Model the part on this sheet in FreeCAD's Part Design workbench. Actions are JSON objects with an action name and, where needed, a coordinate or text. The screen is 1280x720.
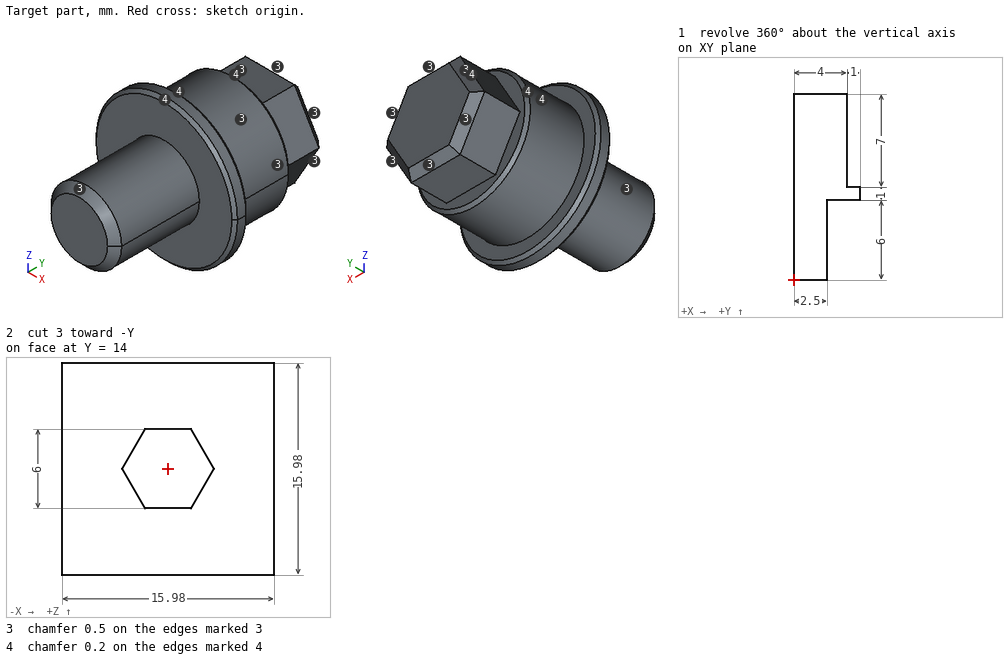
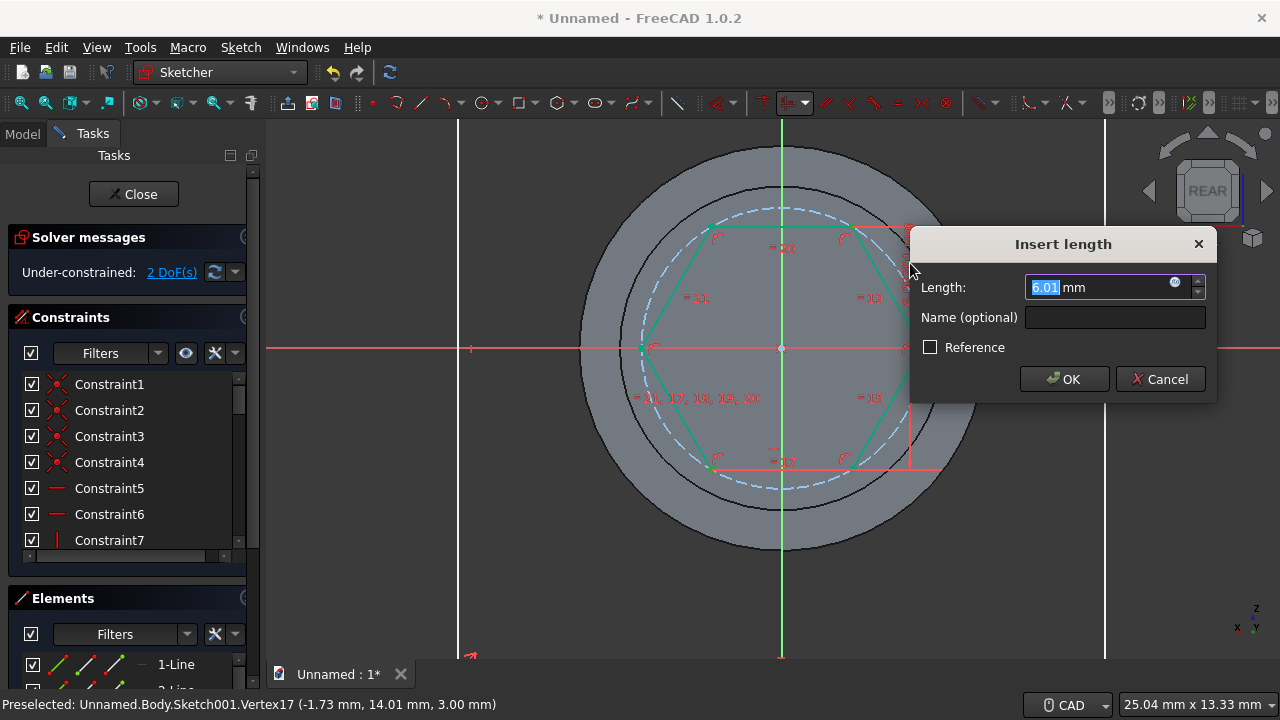
{"action": "type", "text": "6"}
{"action": "key", "text": "Return"}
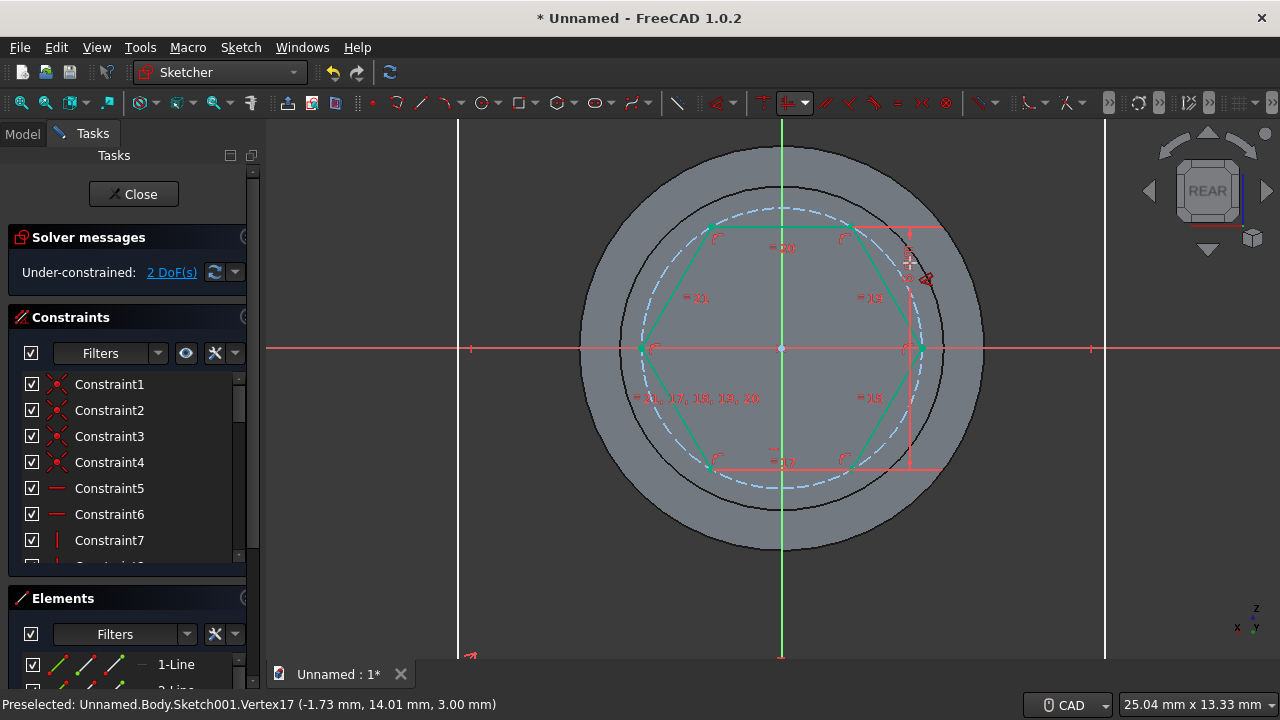
{"action": "scroll", "coordinate": [610, 438], "scroll_direction": "down", "scroll_amount": 3}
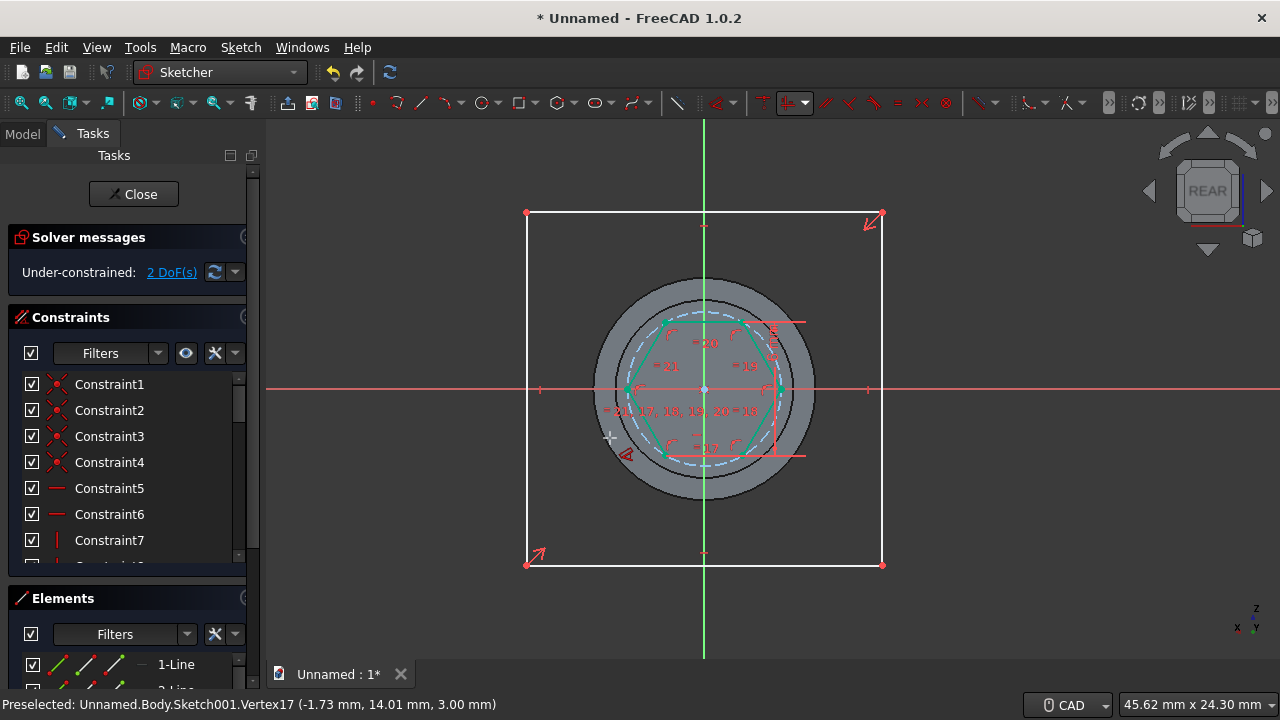
{"action": "left_click", "coordinate": [633, 566]}
{"action": "left_click", "coordinate": [623, 600]}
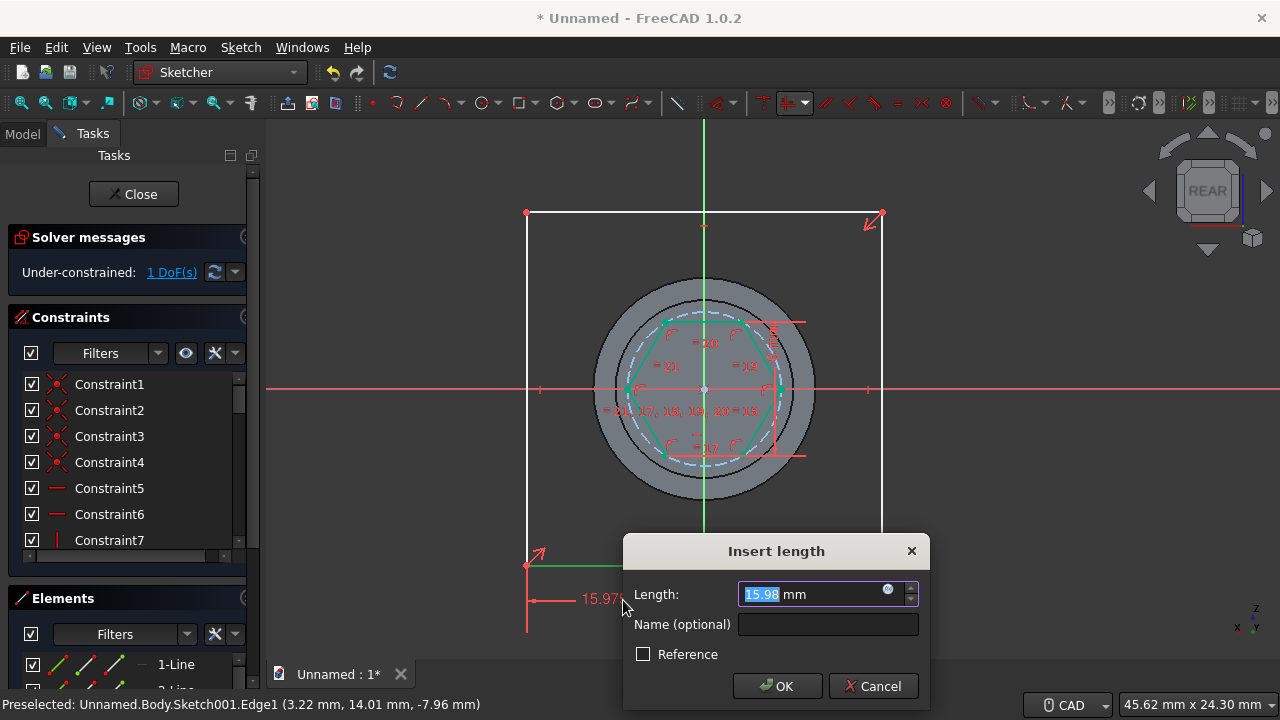
{"action": "type", "text": "15.98"}
{"action": "key", "text": "Return"}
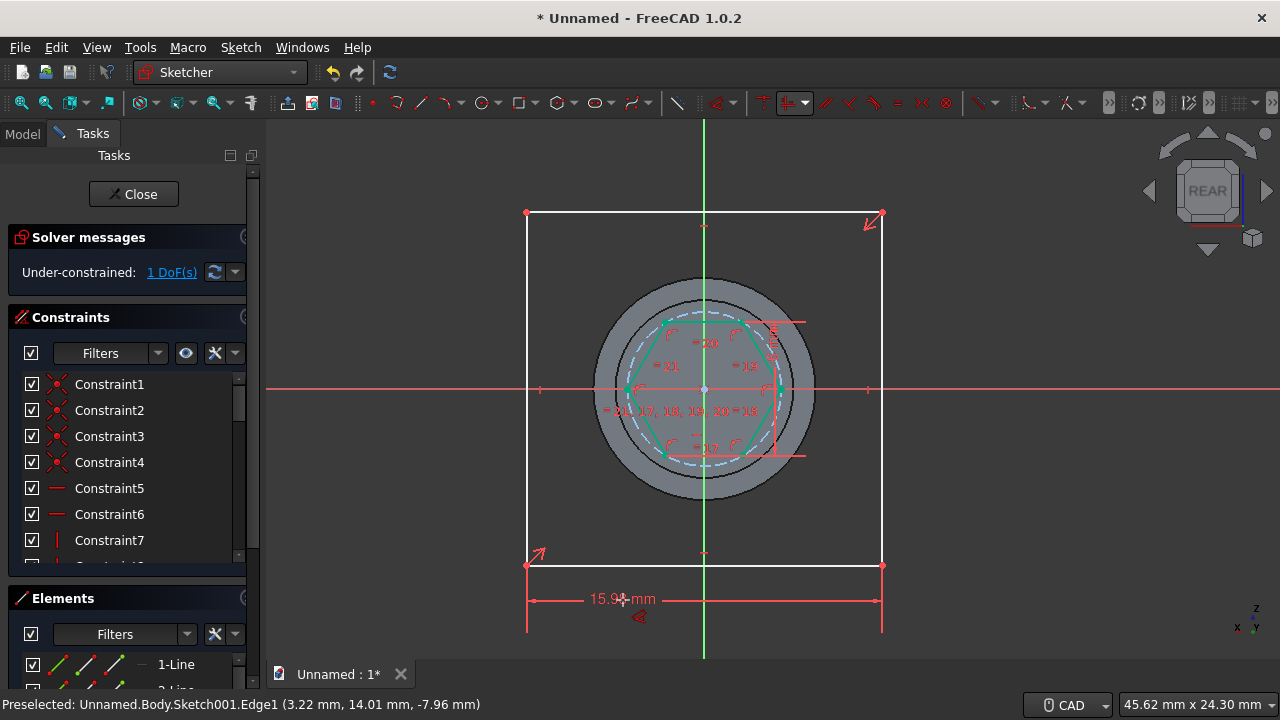
{"action": "left_click", "coordinate": [882, 460]}
{"action": "left_click", "coordinate": [916, 308]}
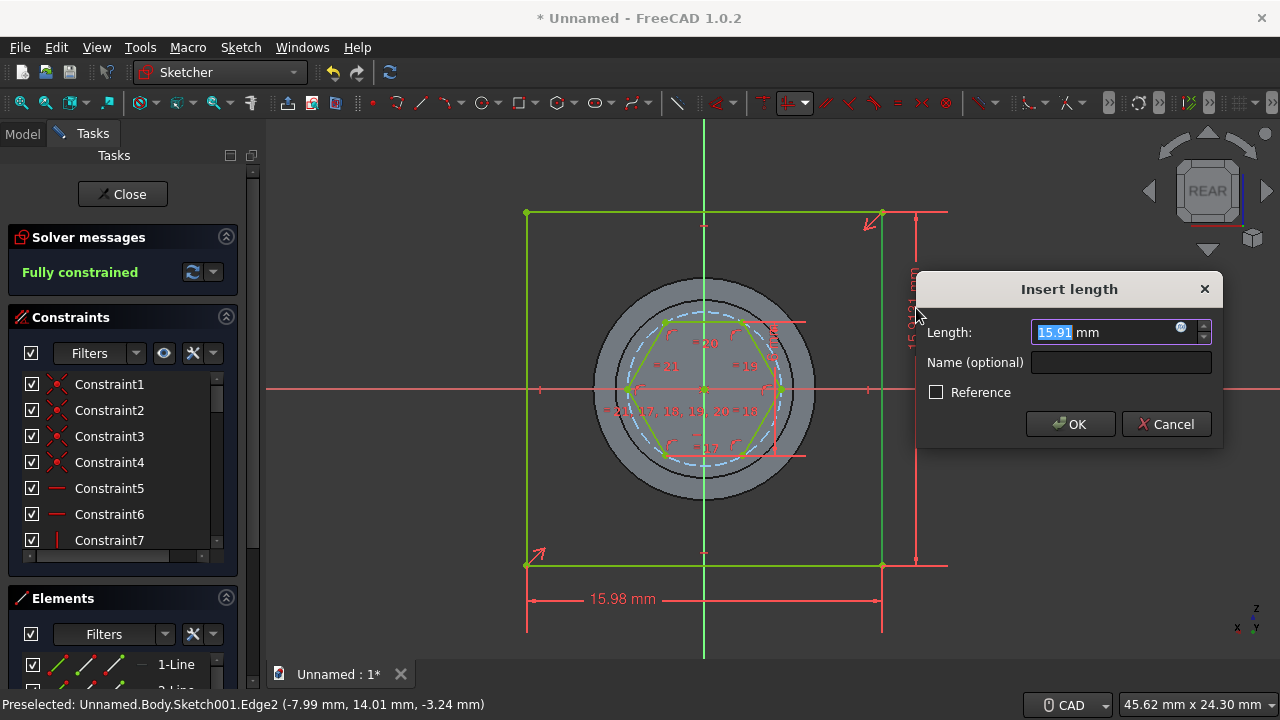
{"action": "type", "text": "15.98"}
{"action": "key", "text": "Return"}
{"action": "key", "text": "Escape"}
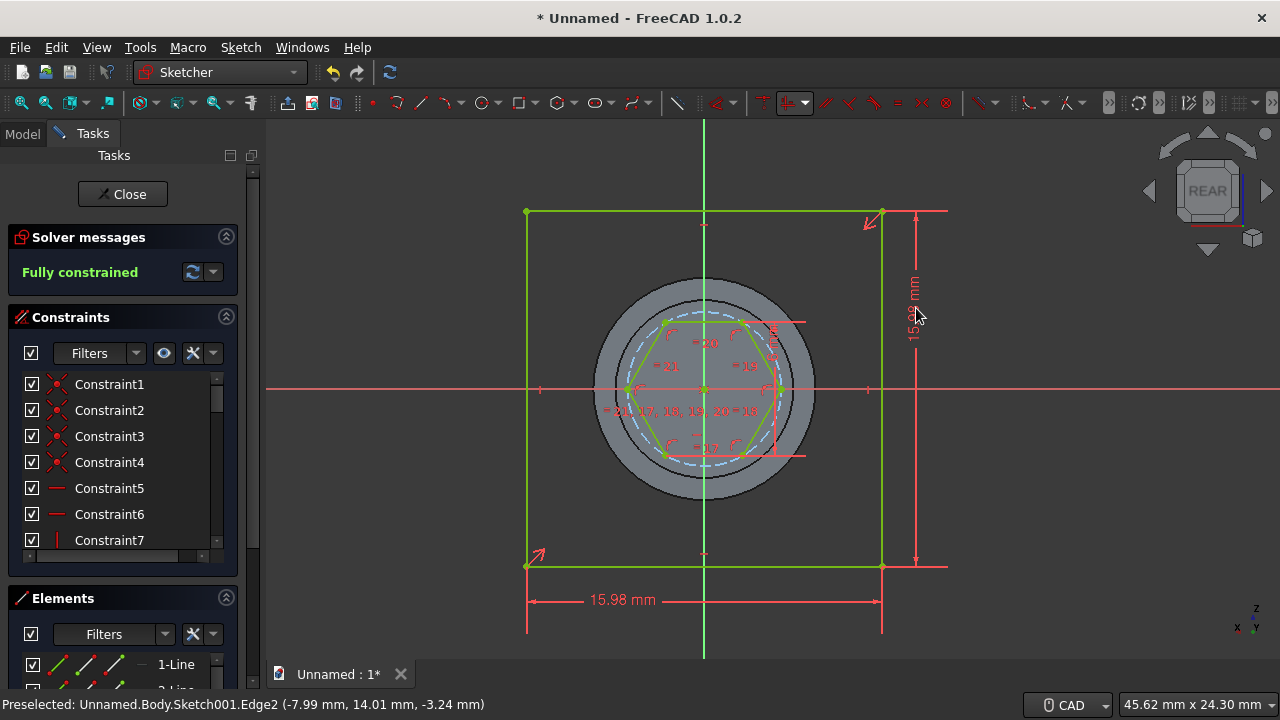
{"action": "left_click", "coordinate": [123, 194]}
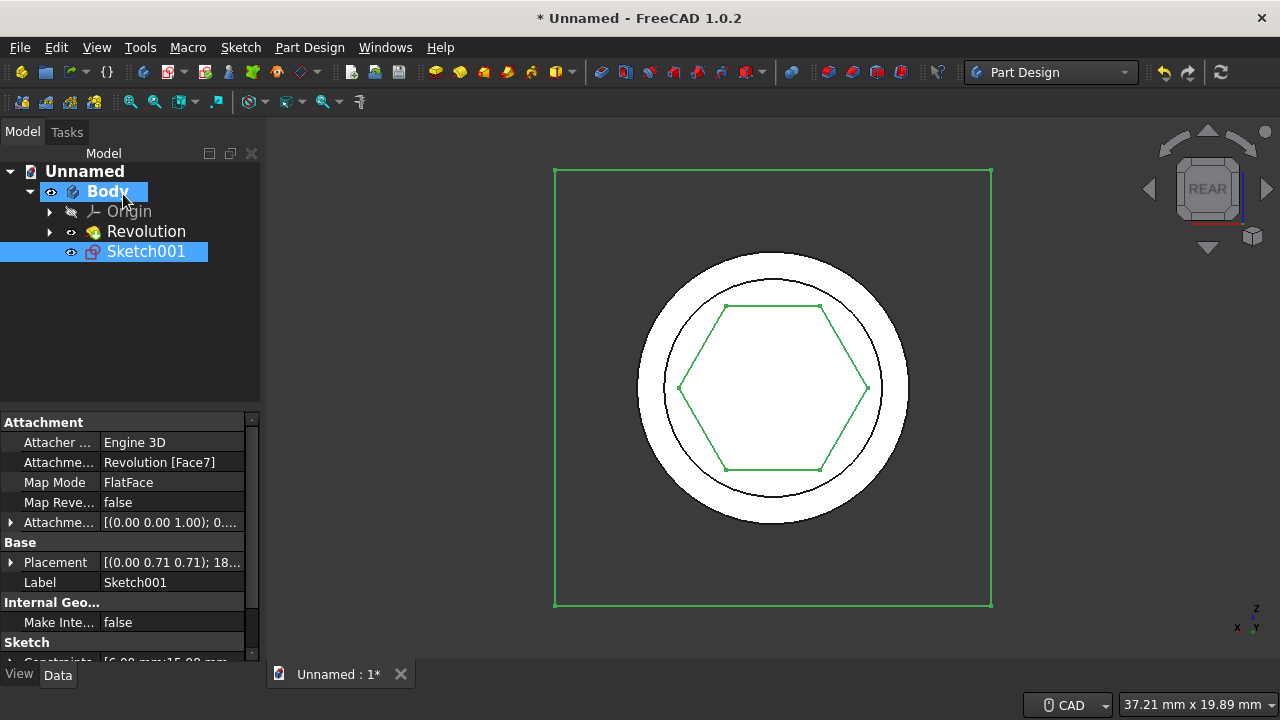
{"action": "left_click", "coordinate": [602, 72]}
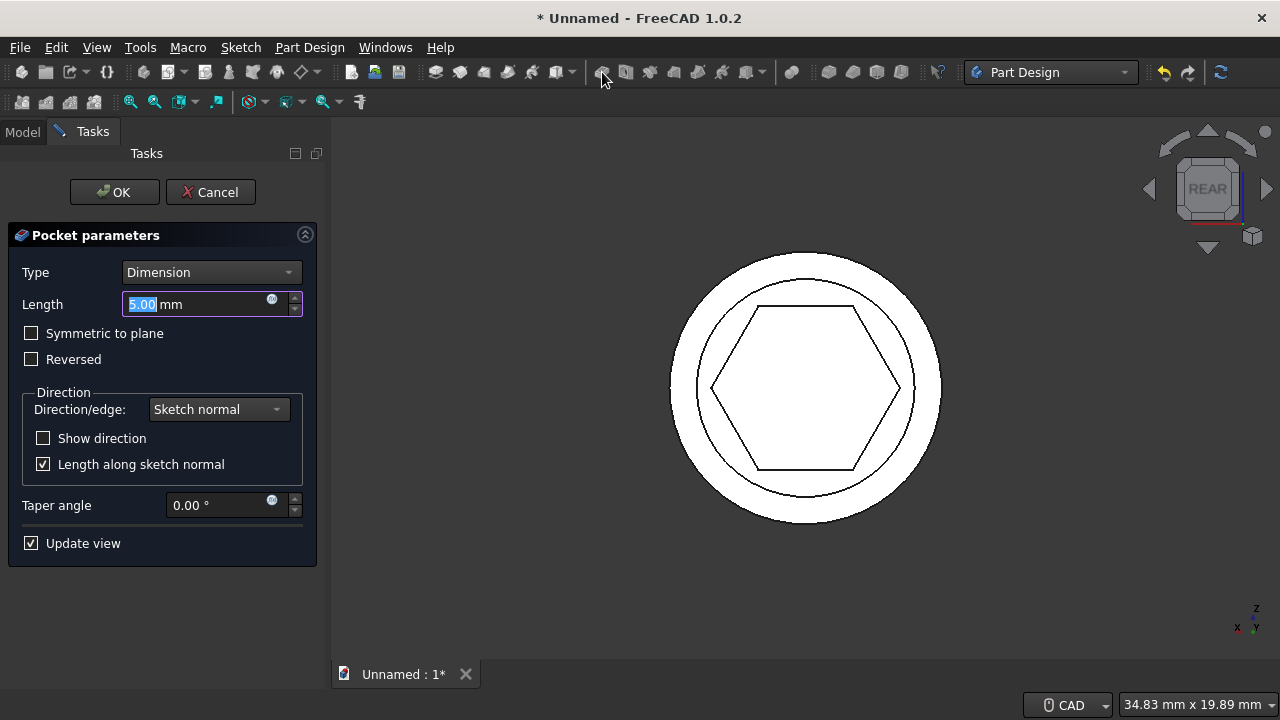
{"action": "type", "text": "3"}
{"action": "key", "text": "Tab"}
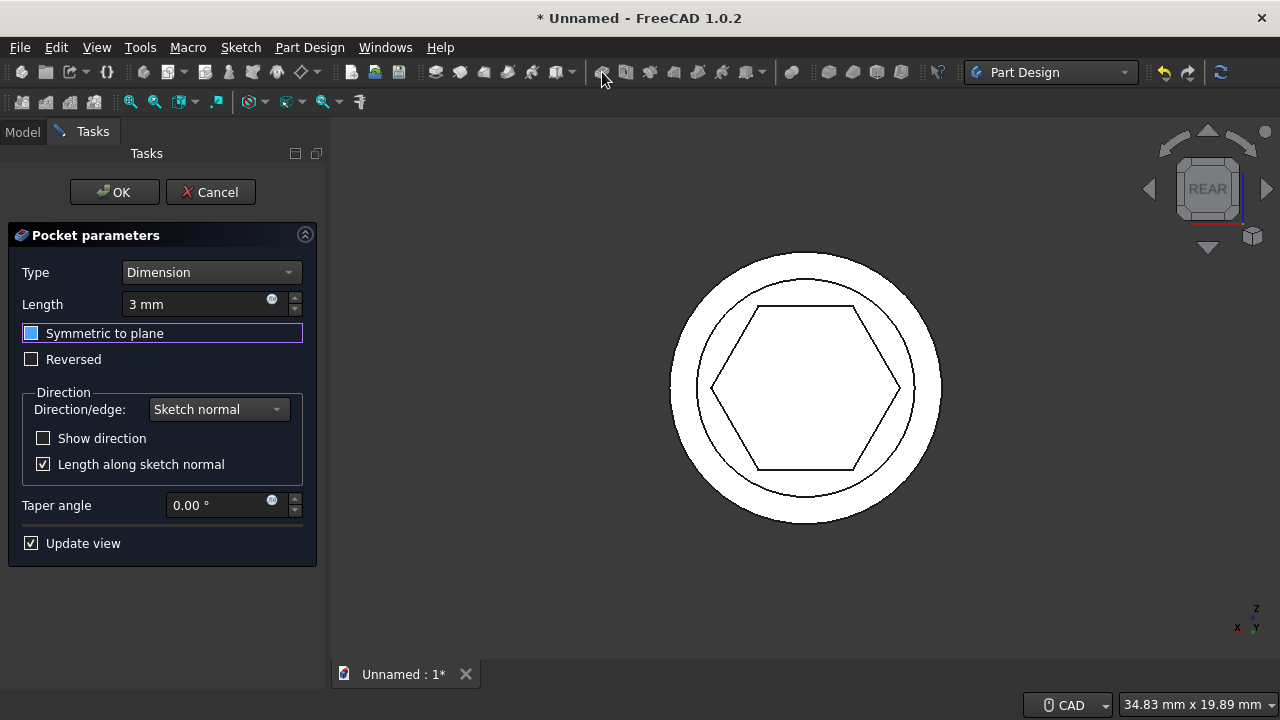
{"action": "left_click", "coordinate": [115, 192]}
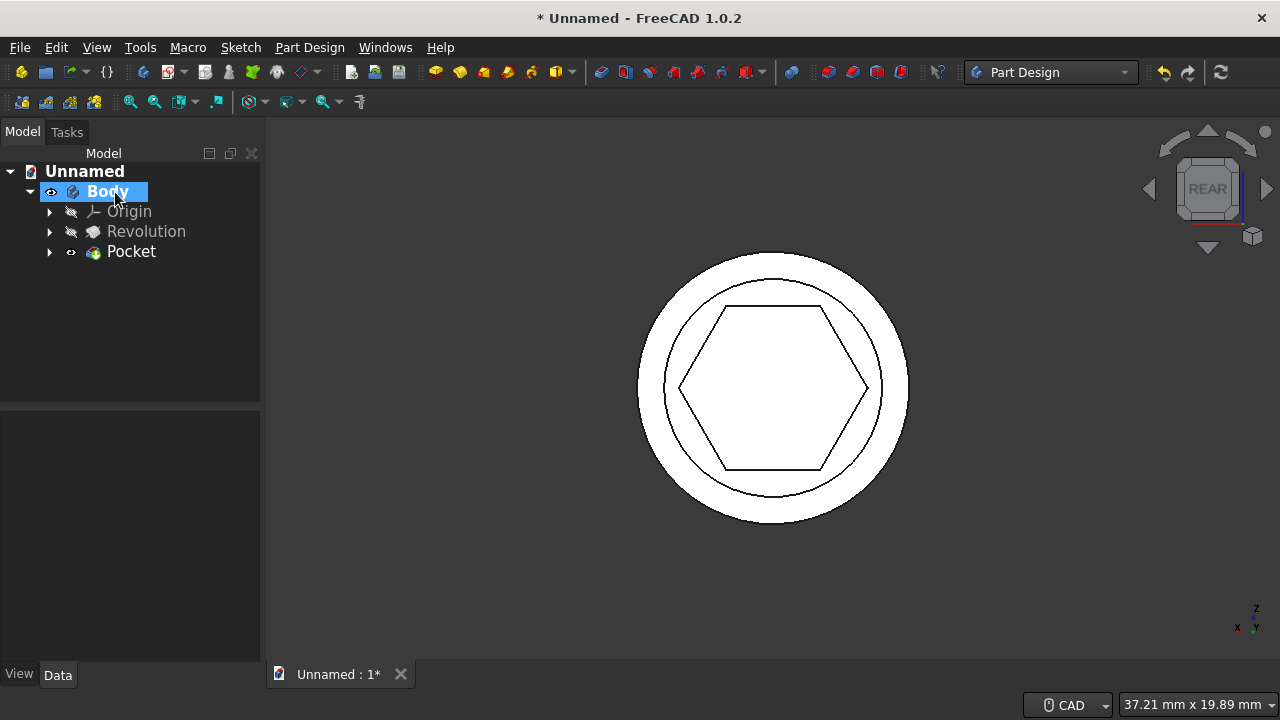
{"action": "left_click", "coordinate": [773, 387]}